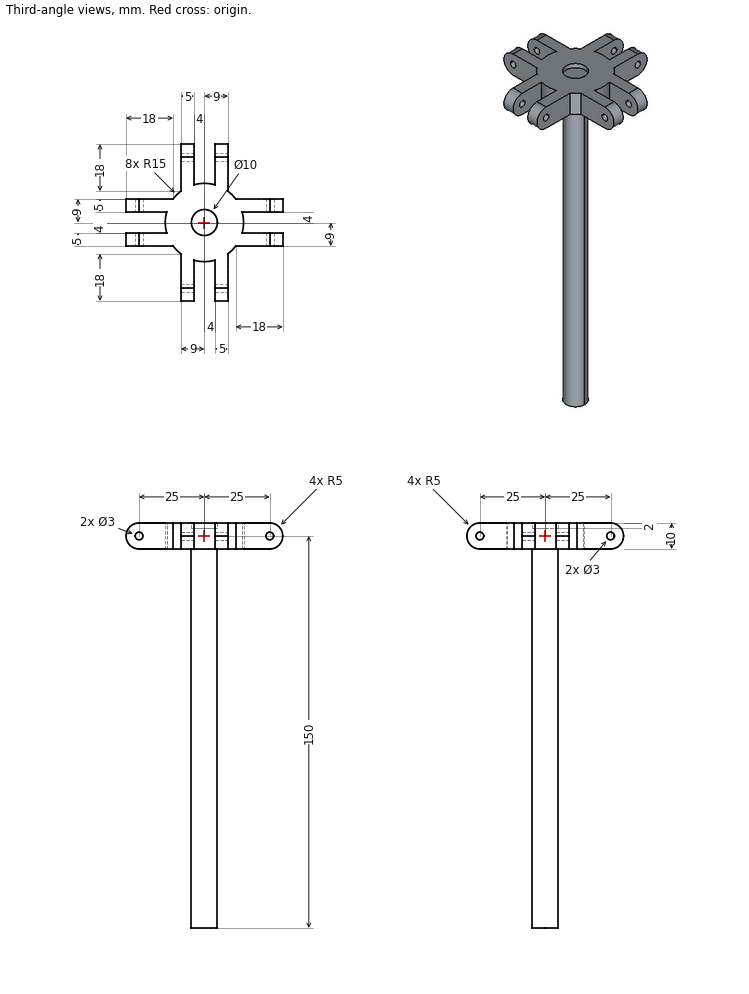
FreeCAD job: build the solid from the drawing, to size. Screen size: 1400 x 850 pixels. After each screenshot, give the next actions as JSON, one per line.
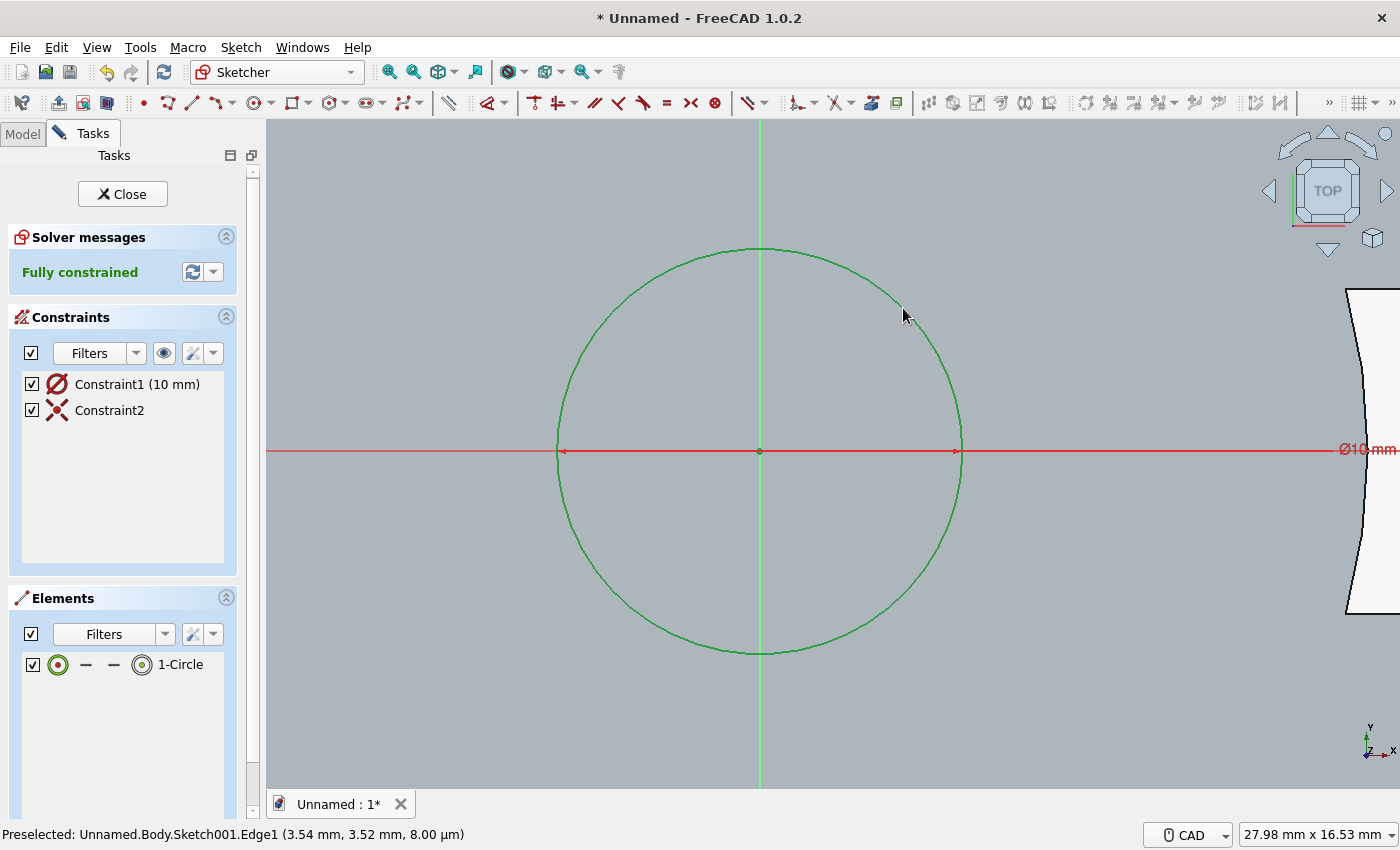
{"action": "left_click", "coordinate": [123, 194]}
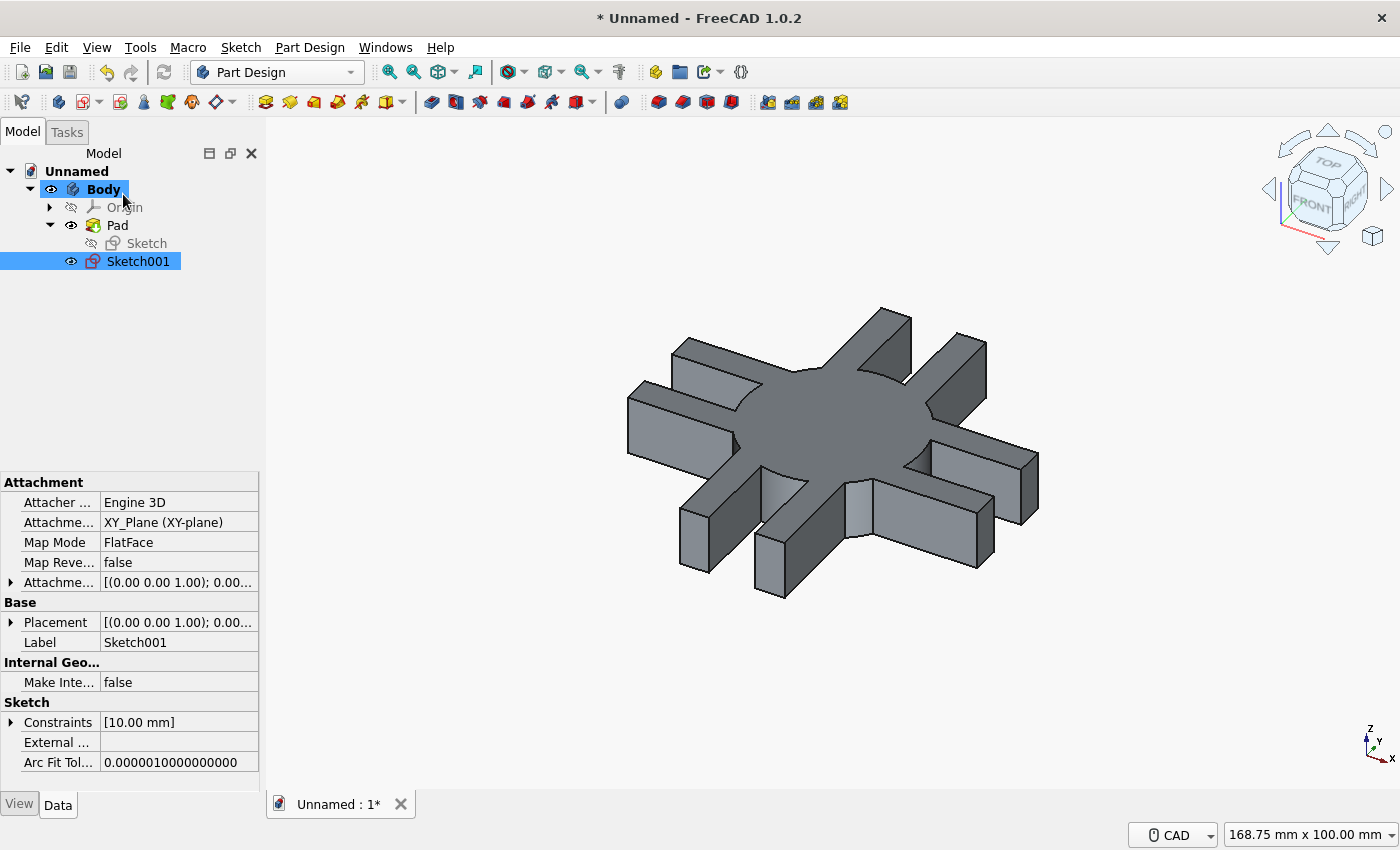
{"action": "left_click", "coordinate": [266, 102]}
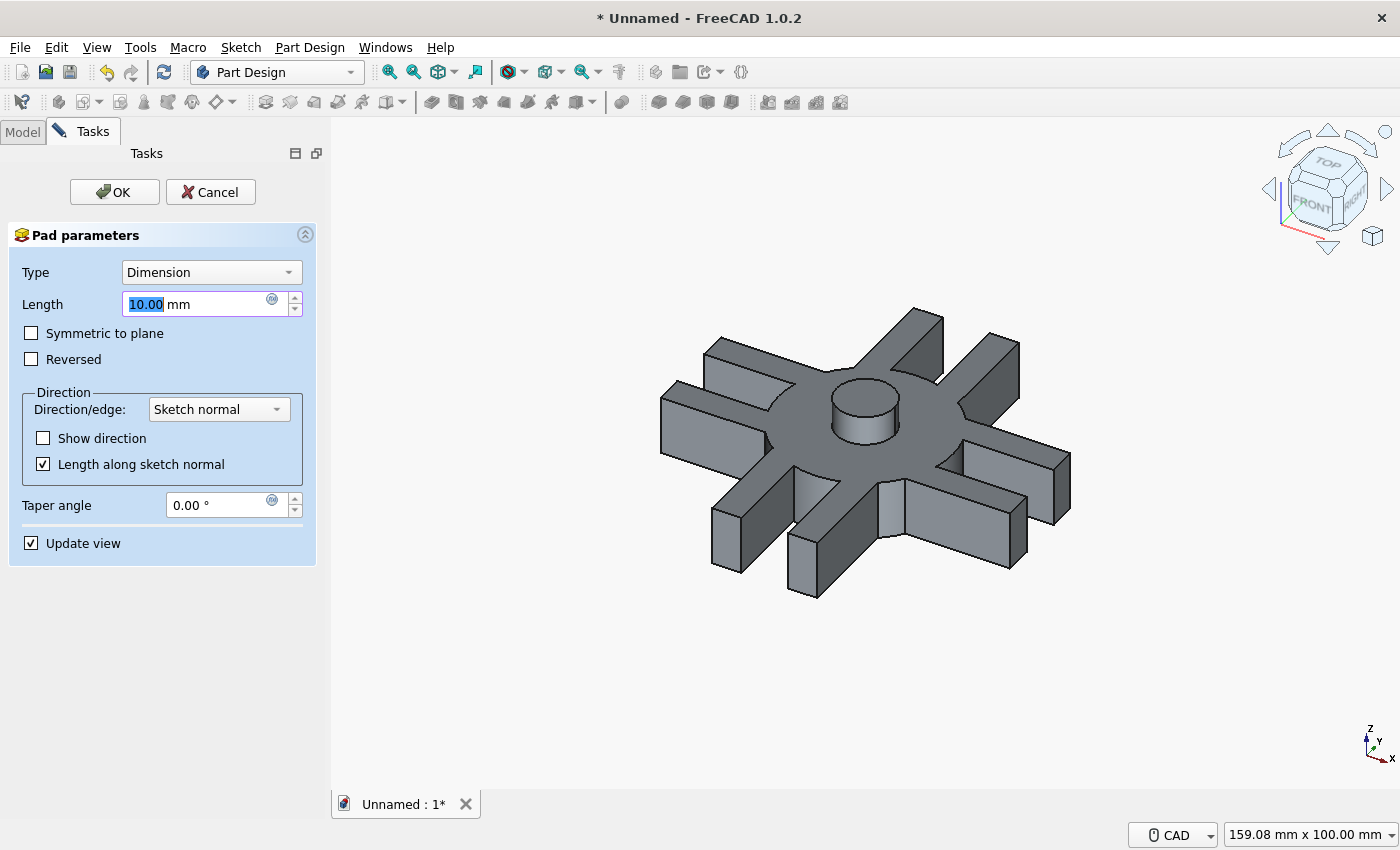
{"action": "type", "text": "150"}
{"action": "key", "text": "Tab"}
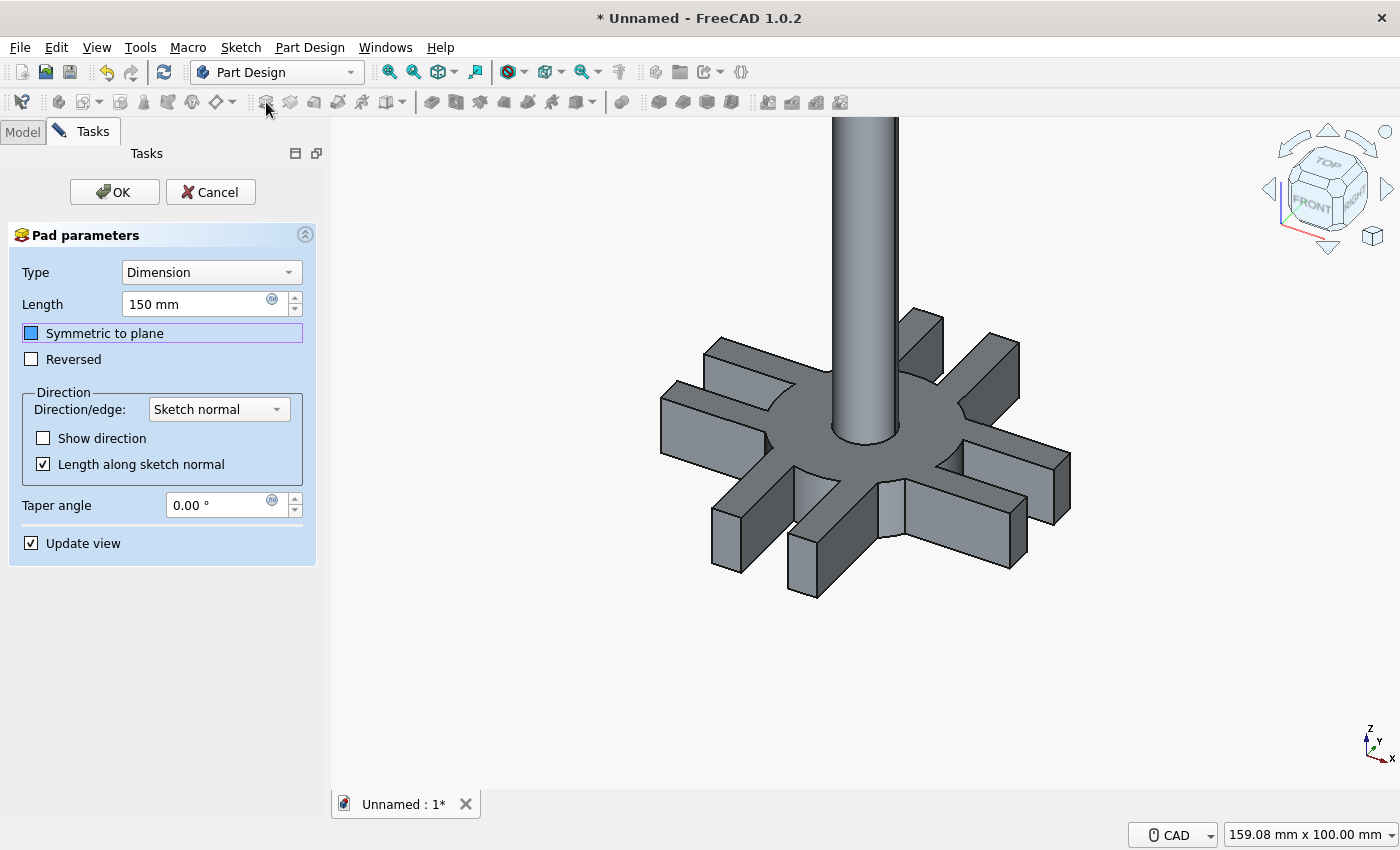
{"action": "left_click", "coordinate": [30, 359]}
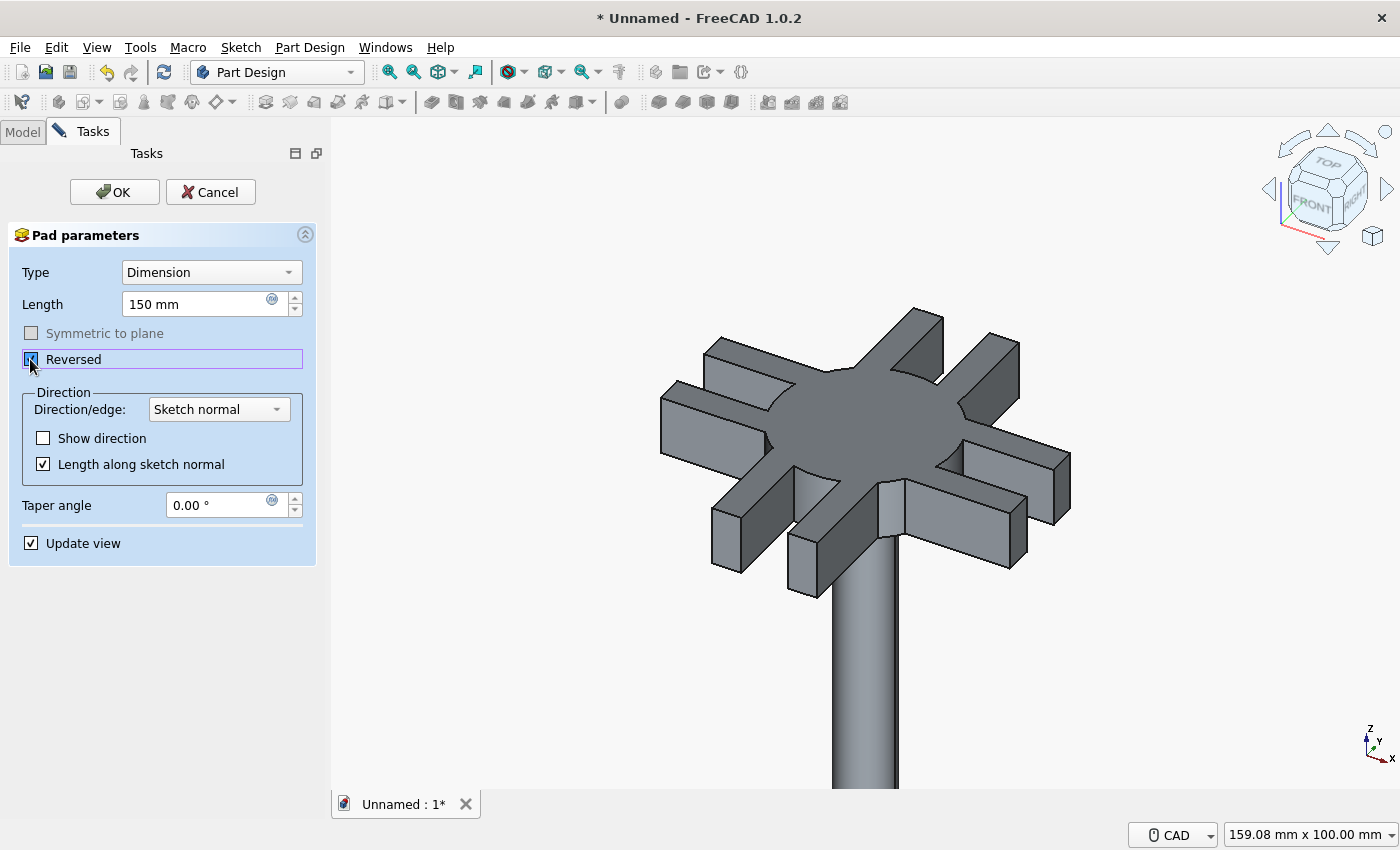
{"action": "left_click", "coordinate": [115, 192]}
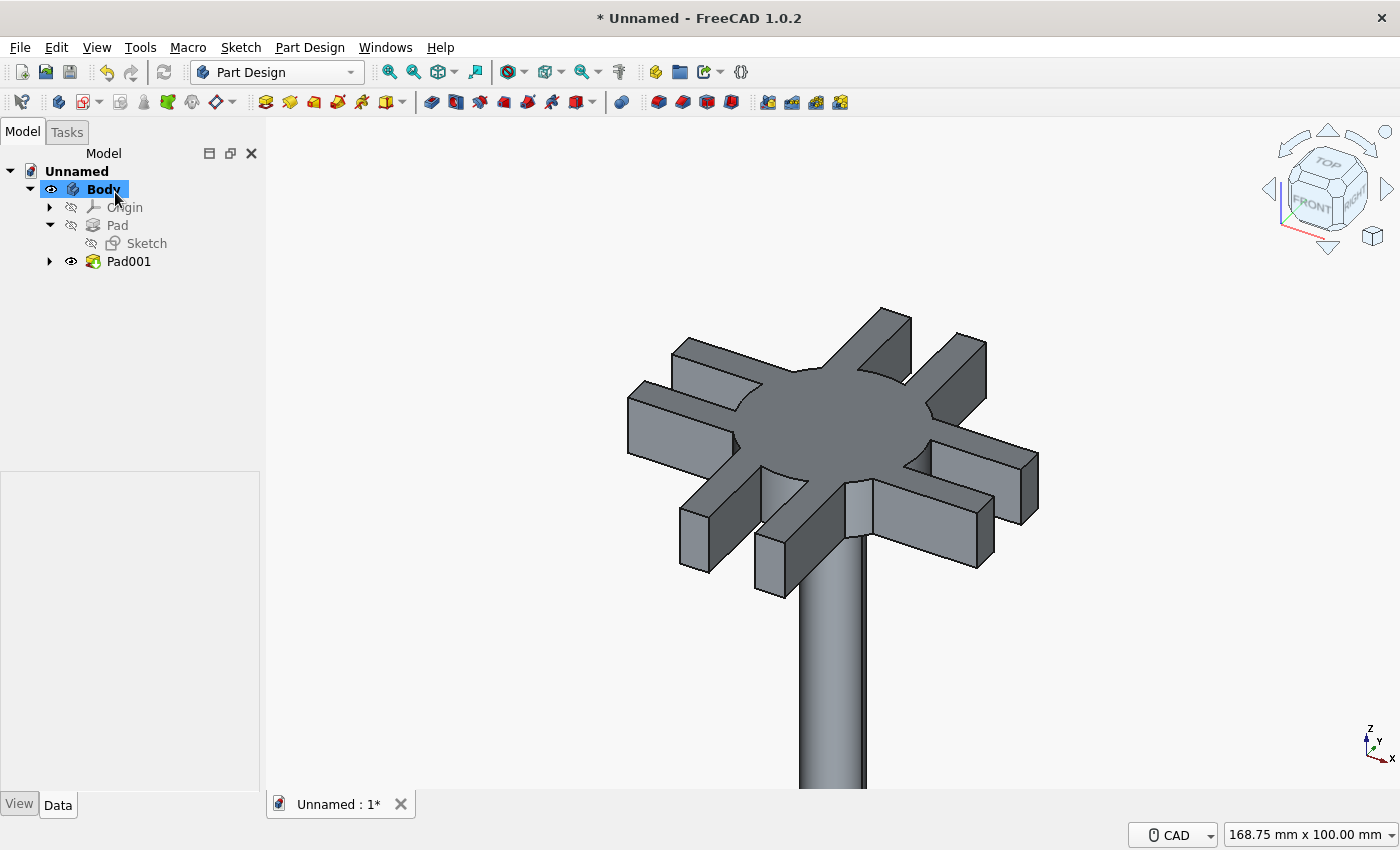
{"action": "key", "text": "v f"}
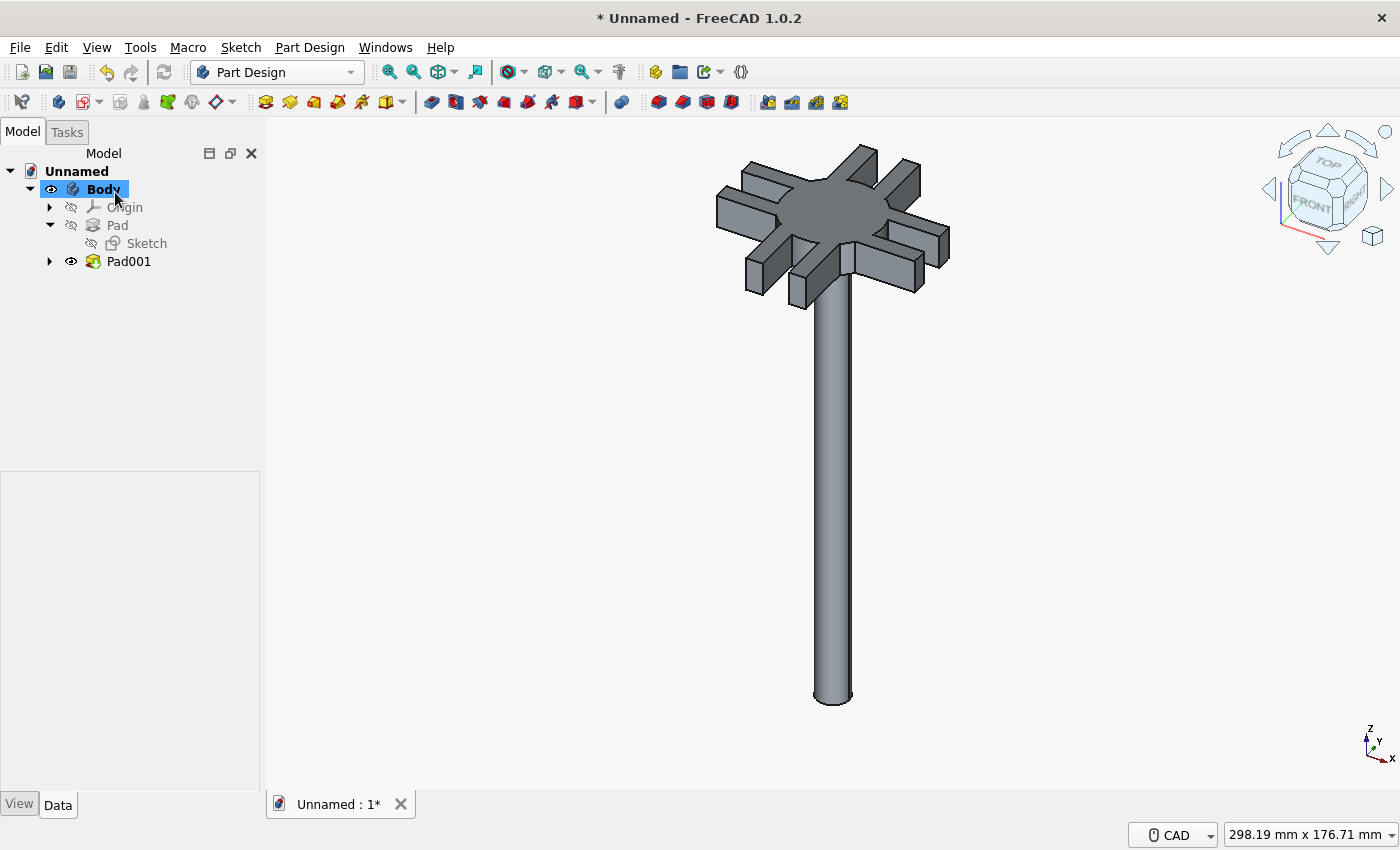
{"action": "left_click", "coordinate": [907, 191]}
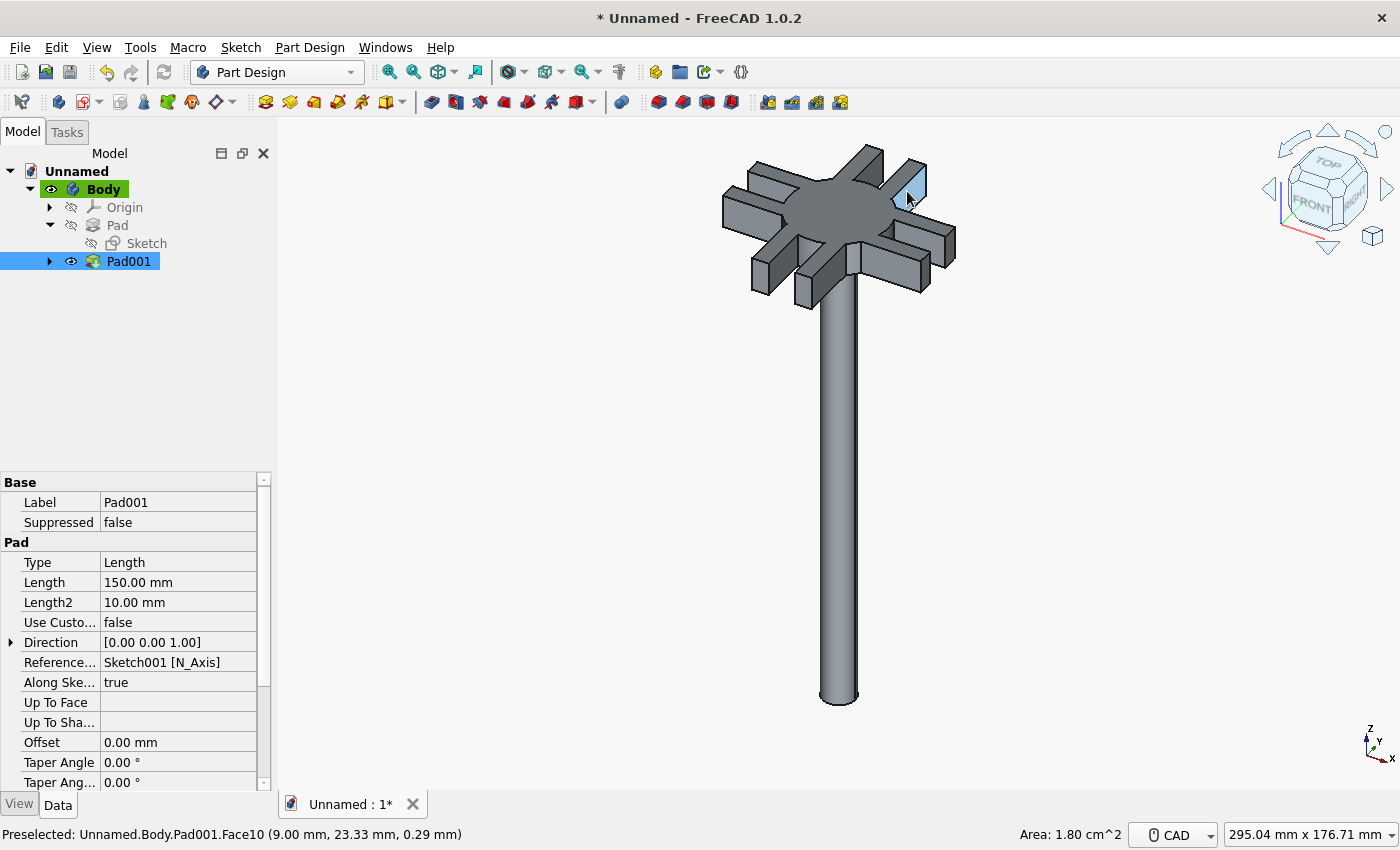
{"action": "left_click", "coordinate": [84, 102]}